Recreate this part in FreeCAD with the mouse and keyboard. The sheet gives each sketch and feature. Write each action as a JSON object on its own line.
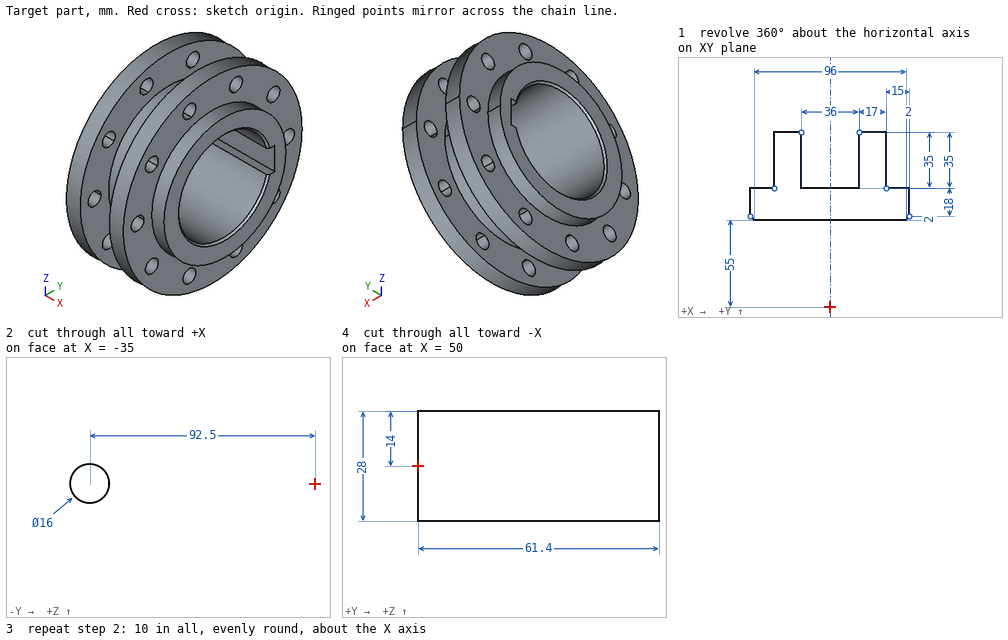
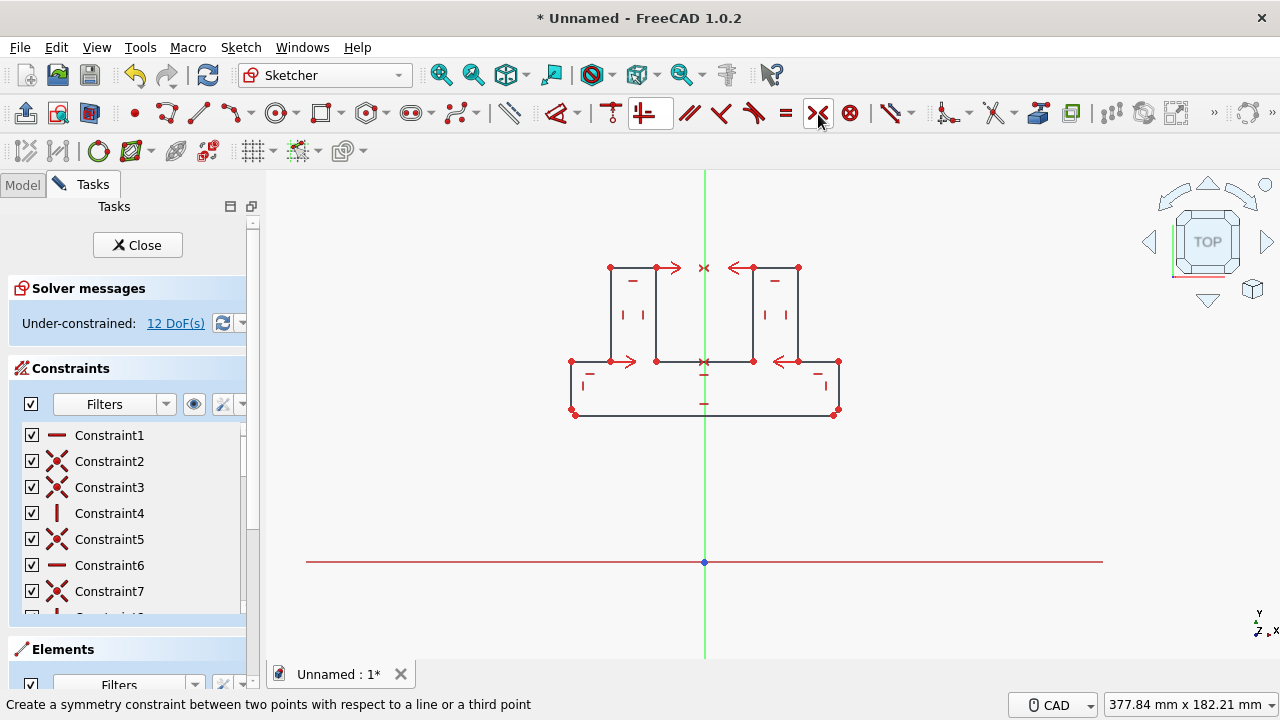
{"action": "scroll", "coordinate": [839, 410], "scroll_direction": "up", "scroll_amount": 3}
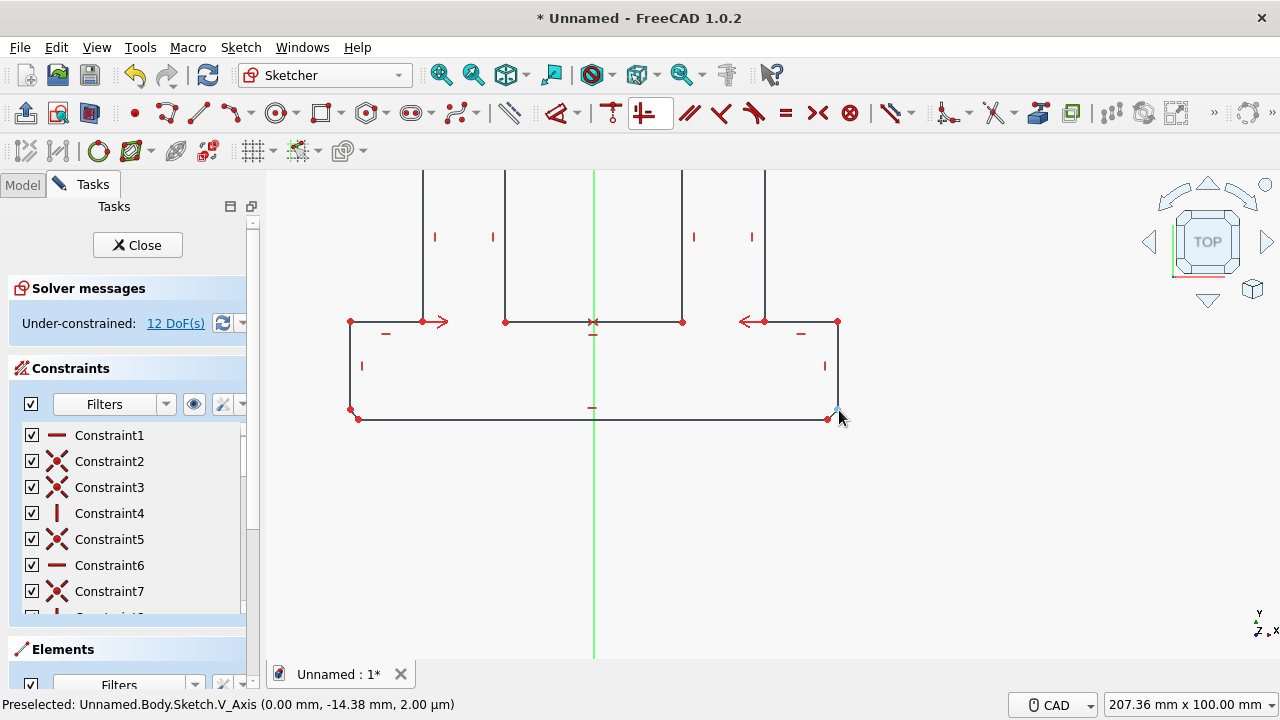
{"action": "left_click", "coordinate": [838, 409]}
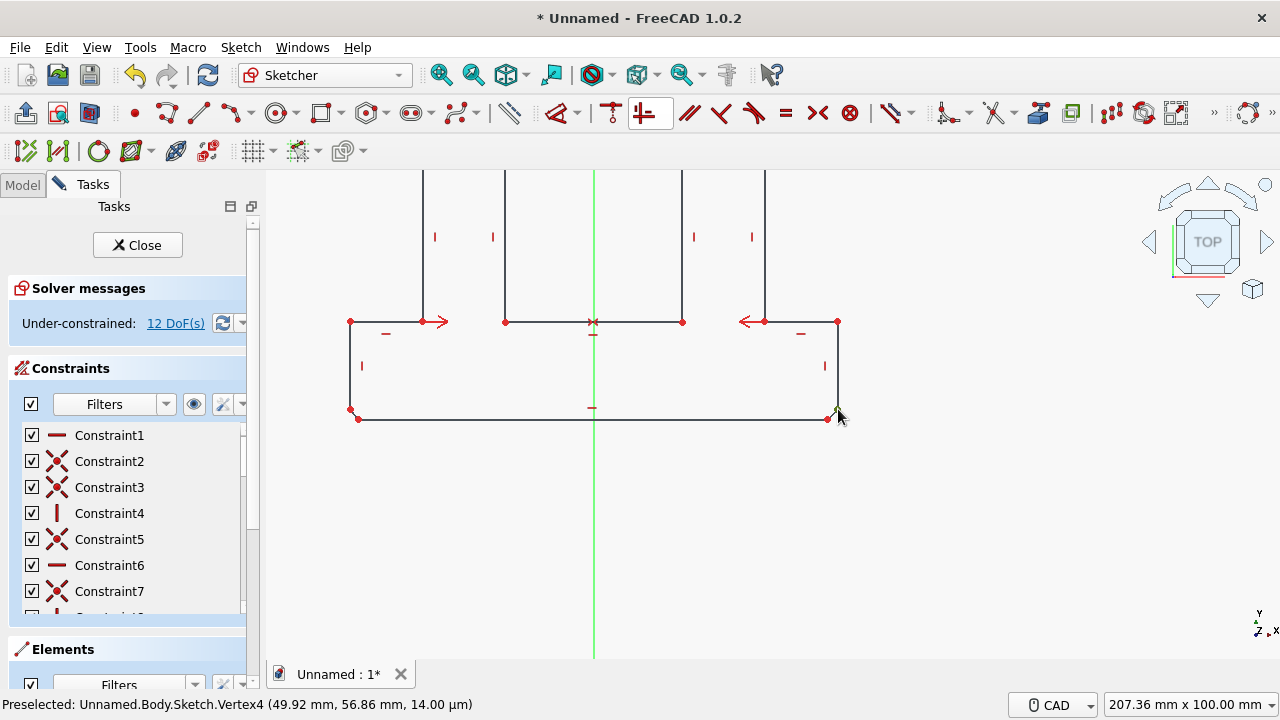
{"action": "left_click", "coordinate": [350, 409]}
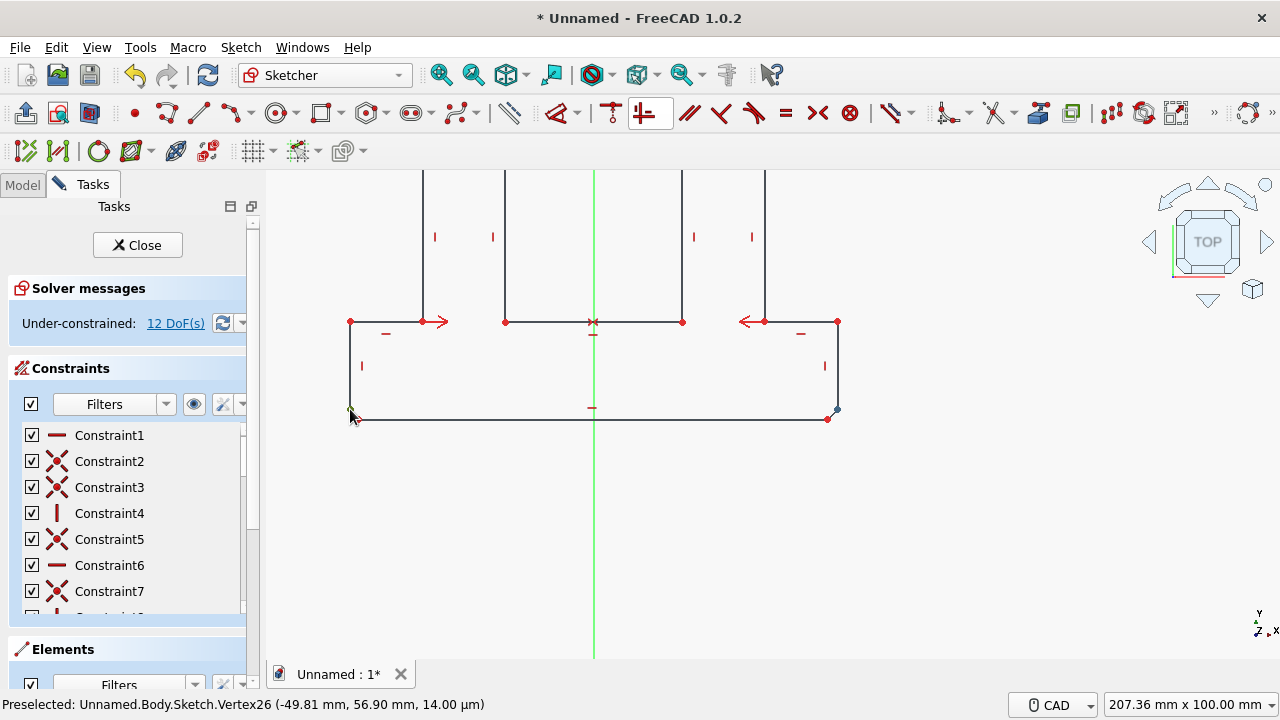
{"action": "left_click", "coordinate": [594, 600]}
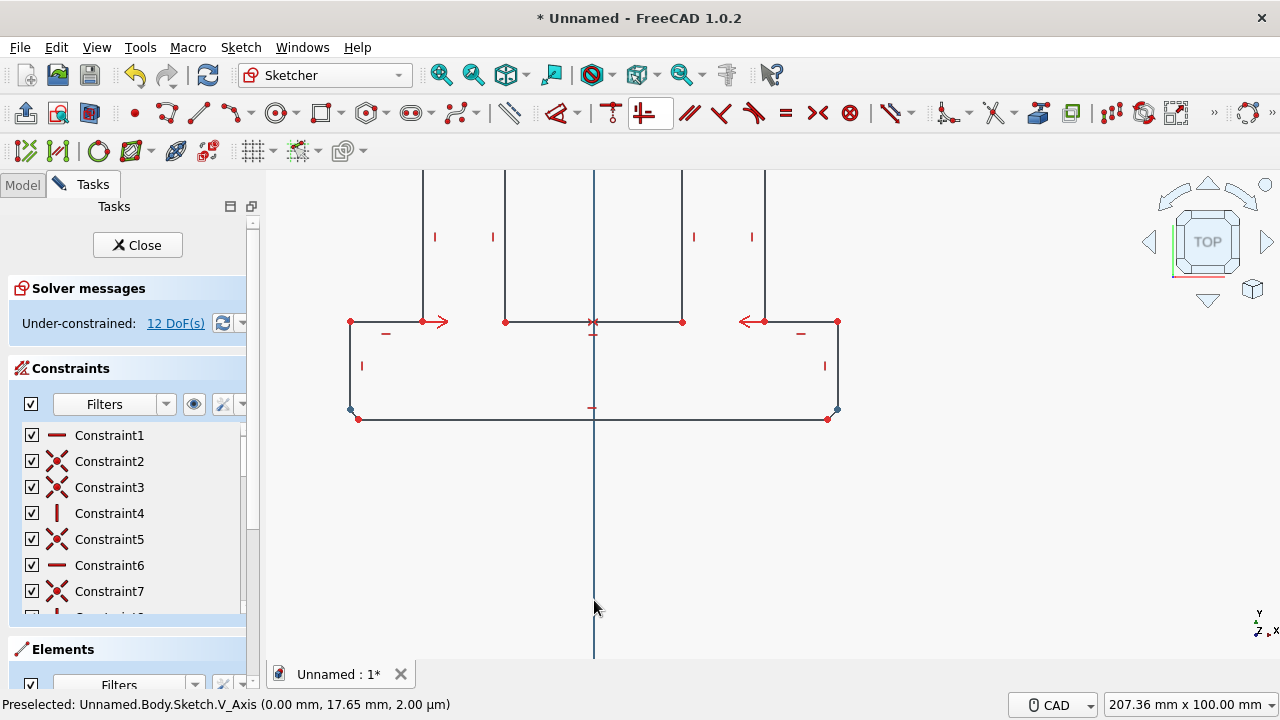
{"action": "left_click", "coordinate": [818, 114]}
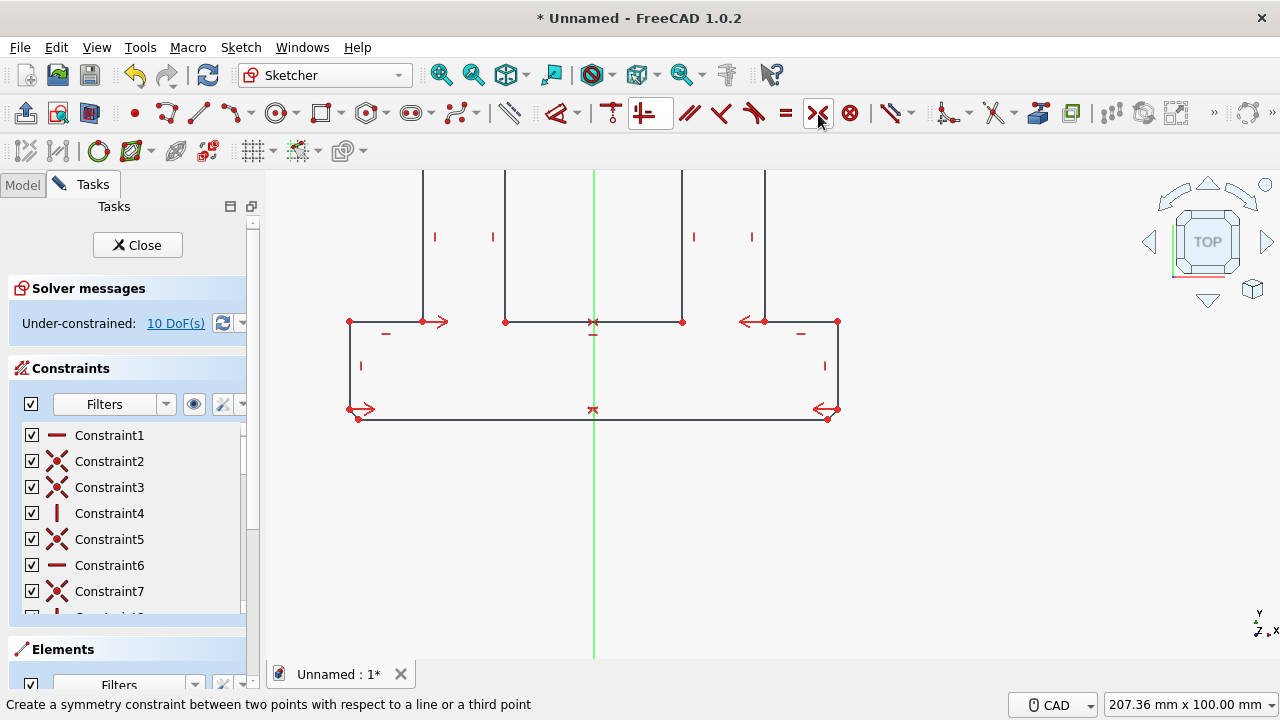
{"action": "left_click", "coordinate": [556, 114]}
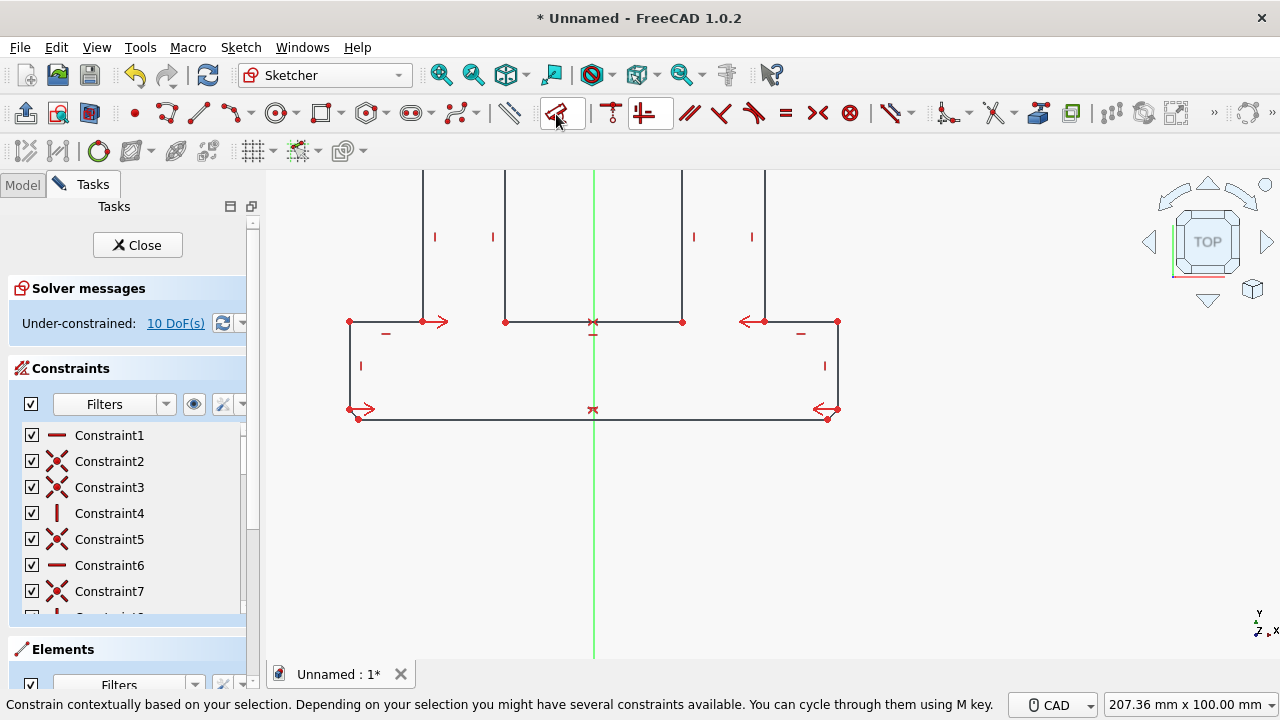
{"action": "left_click", "coordinate": [499, 420]}
{"action": "left_click", "coordinate": [485, 454]}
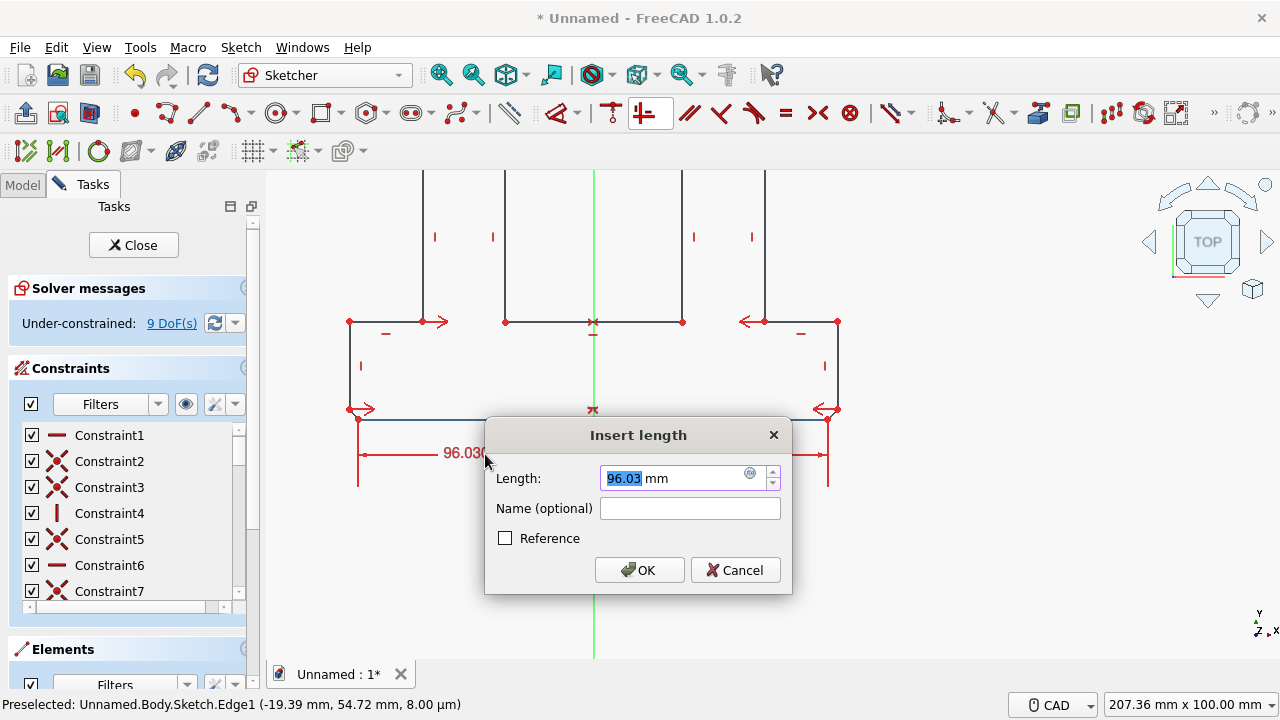
{"action": "type", "text": "96"}
{"action": "key", "text": "Return"}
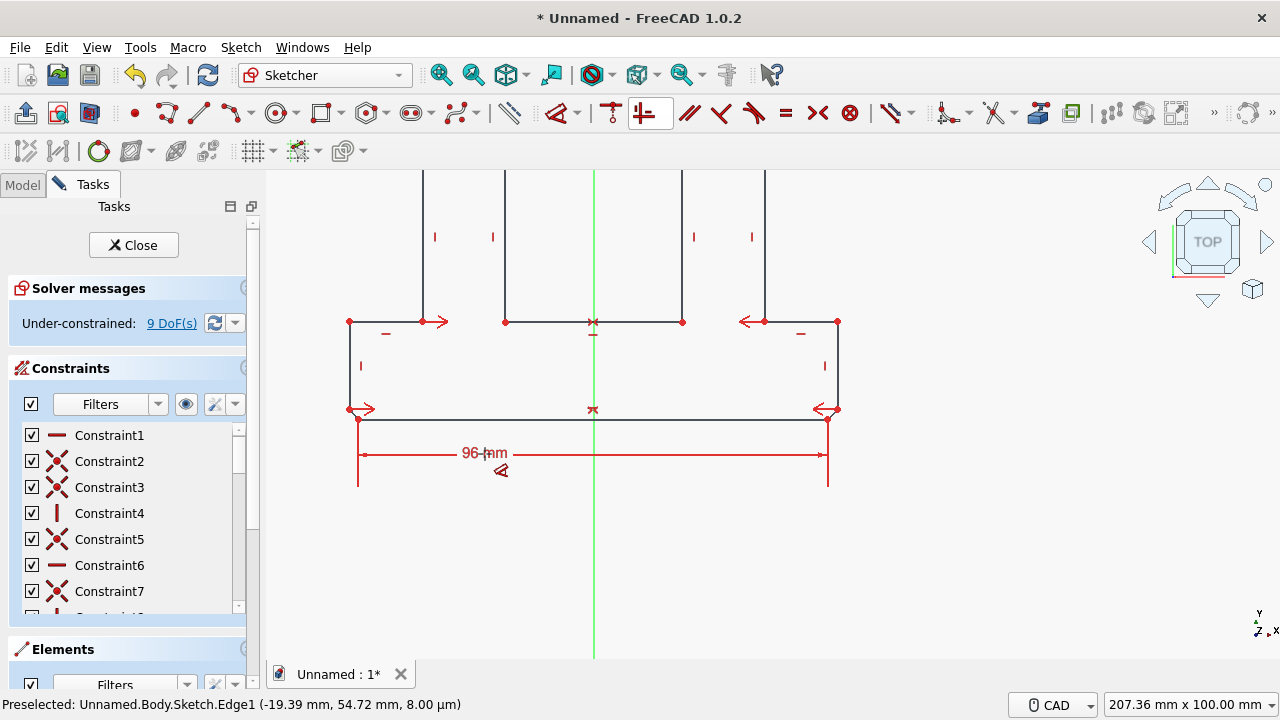
{"action": "left_click", "coordinate": [838, 383]}
{"action": "left_click", "coordinate": [872, 365]}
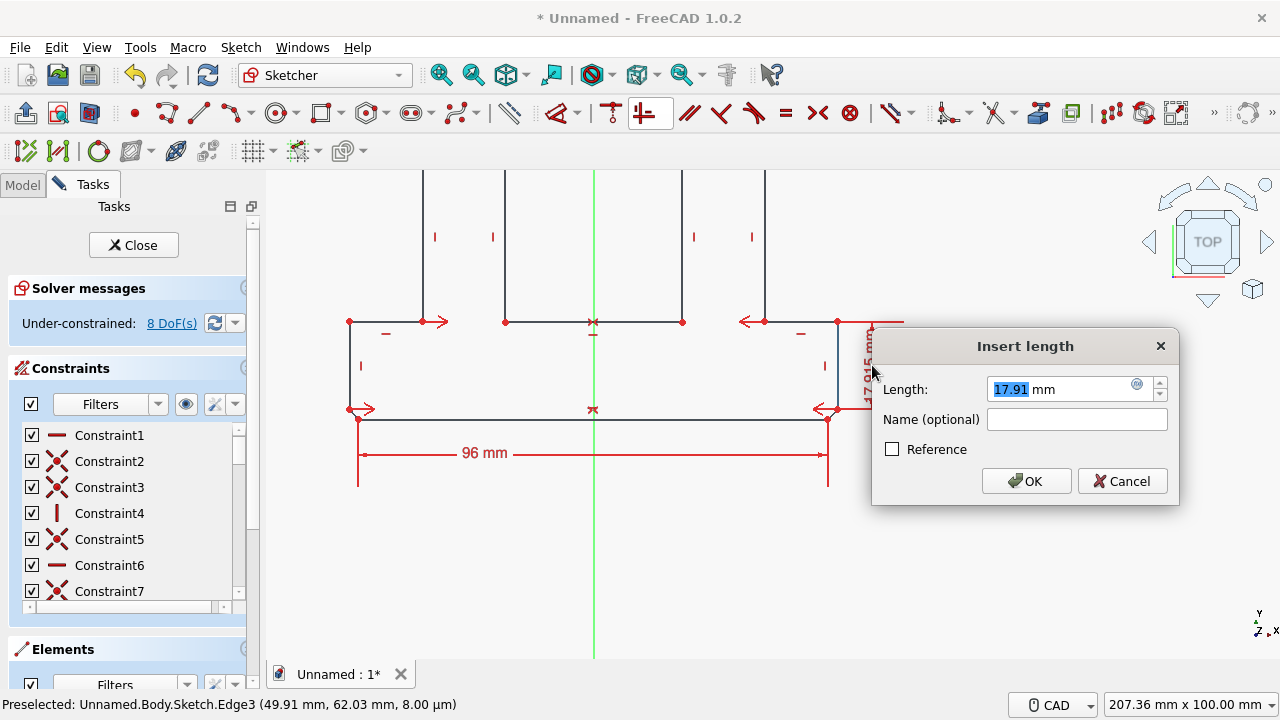
{"action": "type", "text": "18"}
{"action": "key", "text": "Return"}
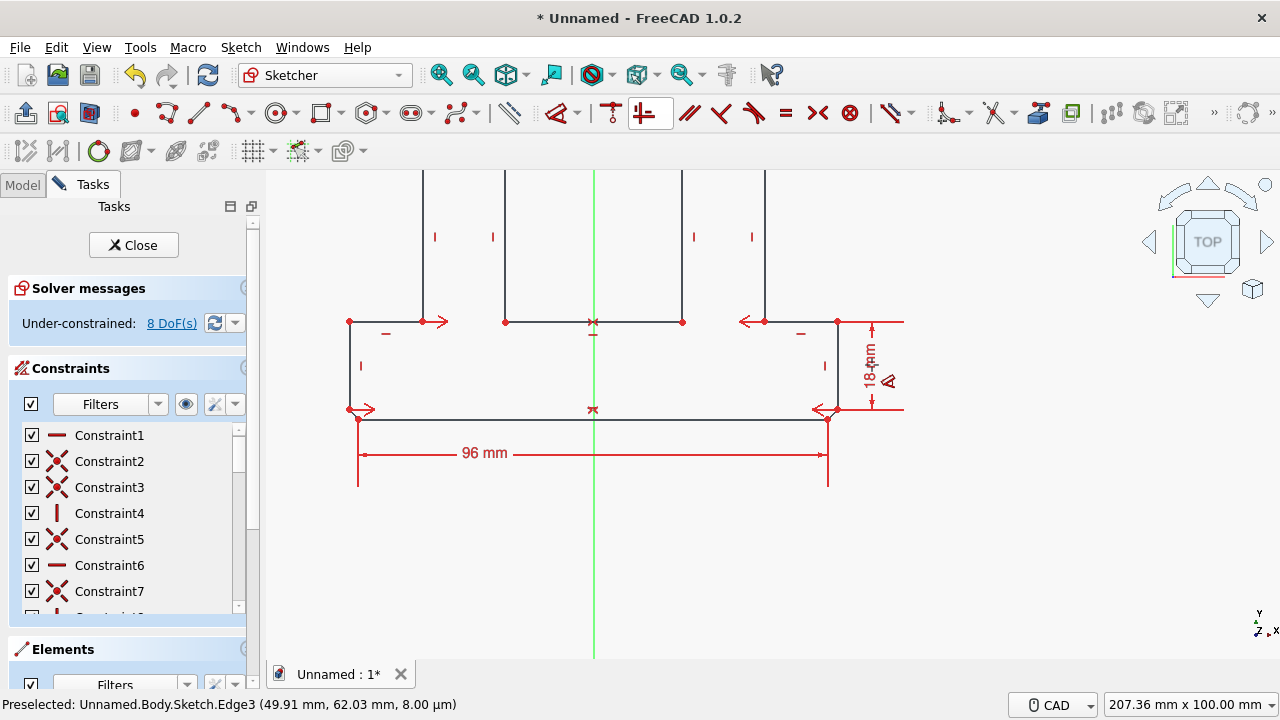
{"action": "left_click", "coordinate": [816, 322]}
{"action": "left_click", "coordinate": [801, 288]}